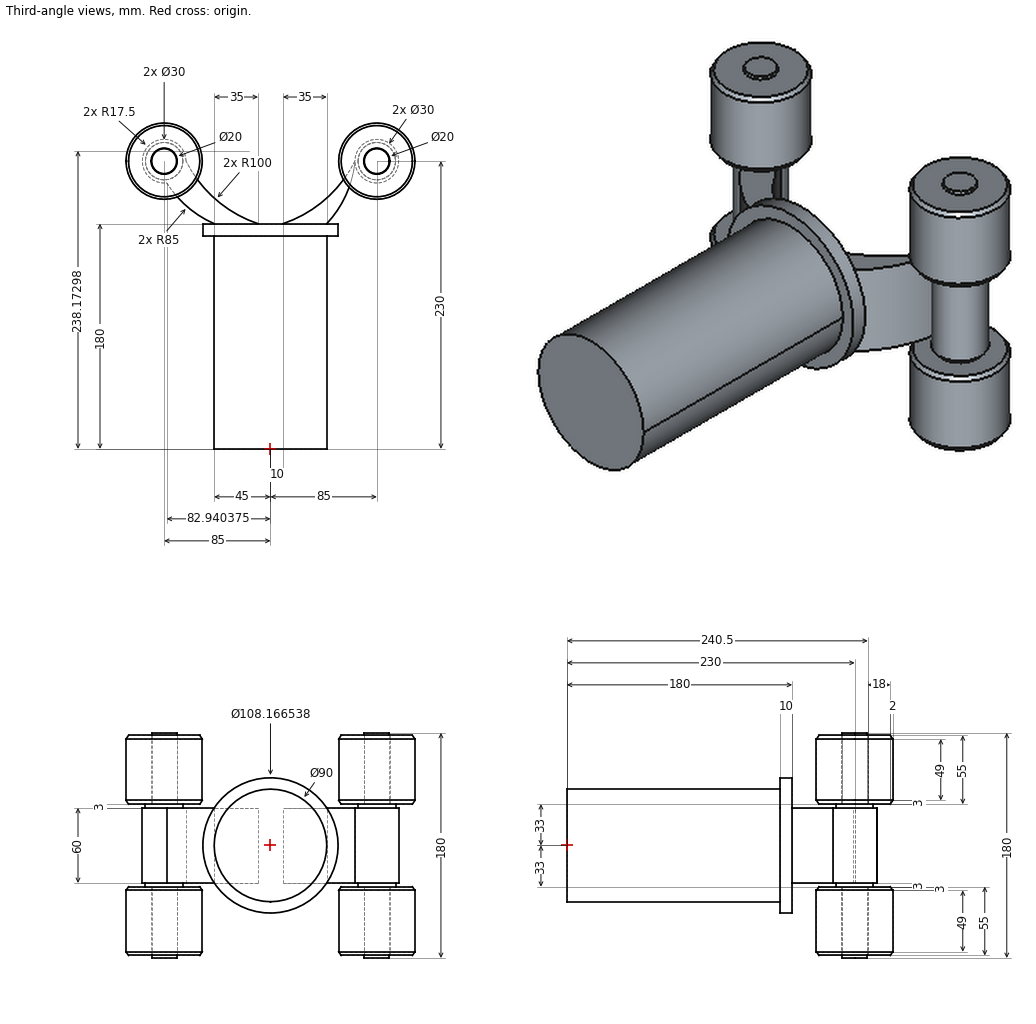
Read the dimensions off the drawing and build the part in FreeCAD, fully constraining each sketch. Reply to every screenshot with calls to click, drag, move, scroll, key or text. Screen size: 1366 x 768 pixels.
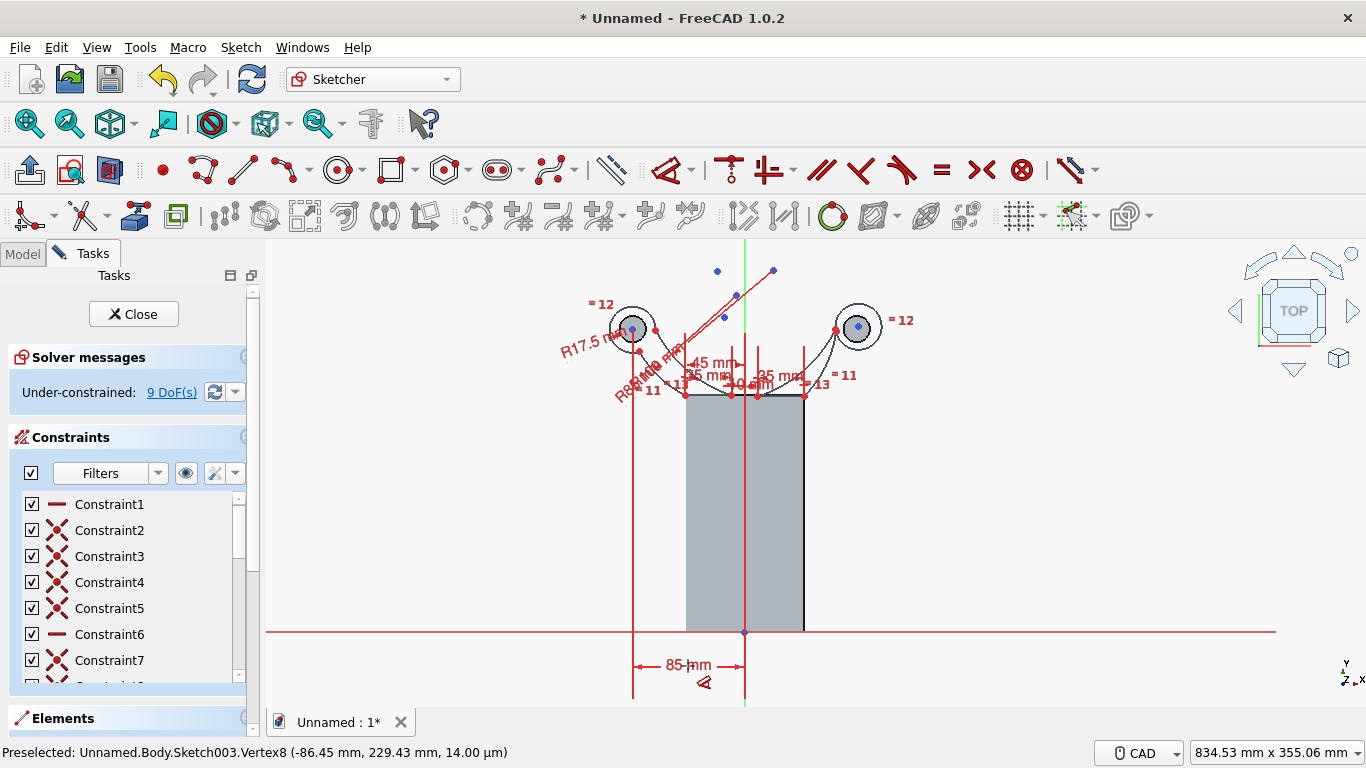
click(859, 327)
click(802, 666)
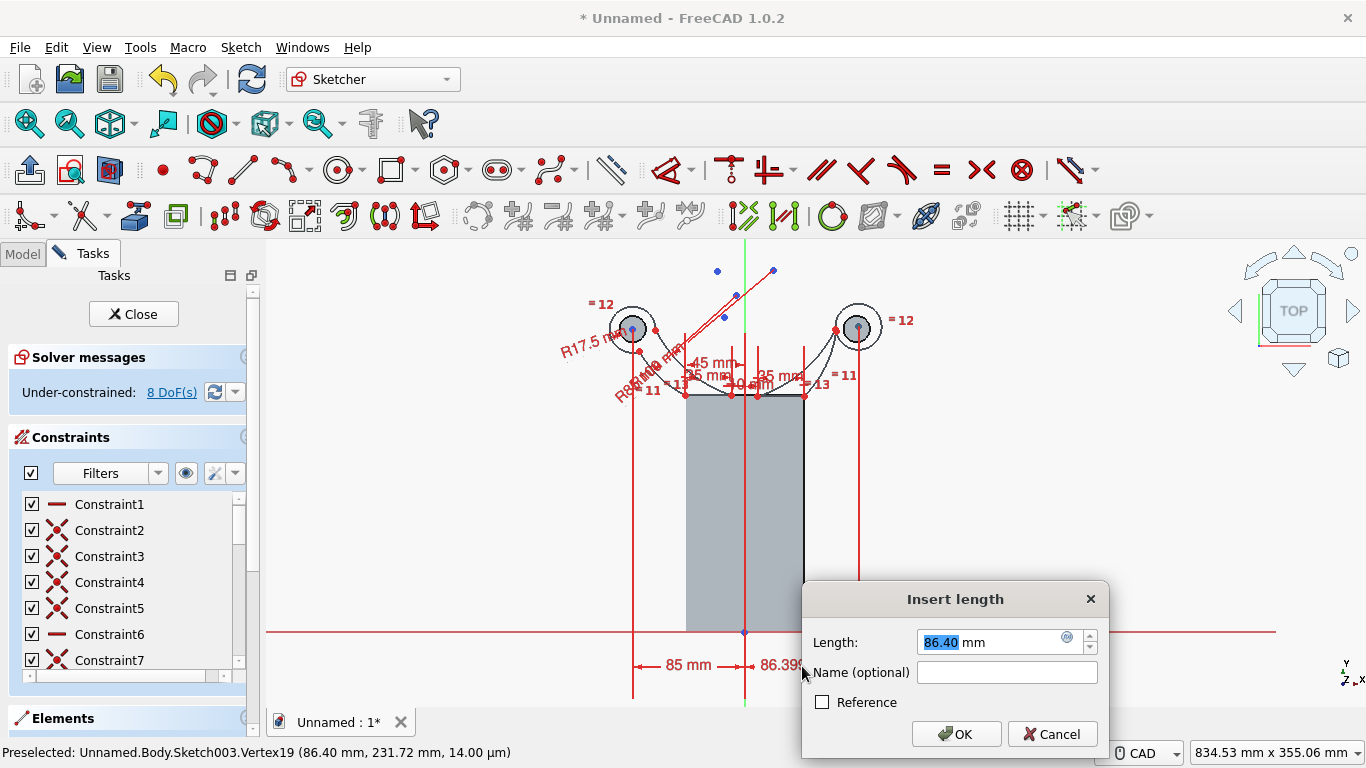
text(85)
key(Return)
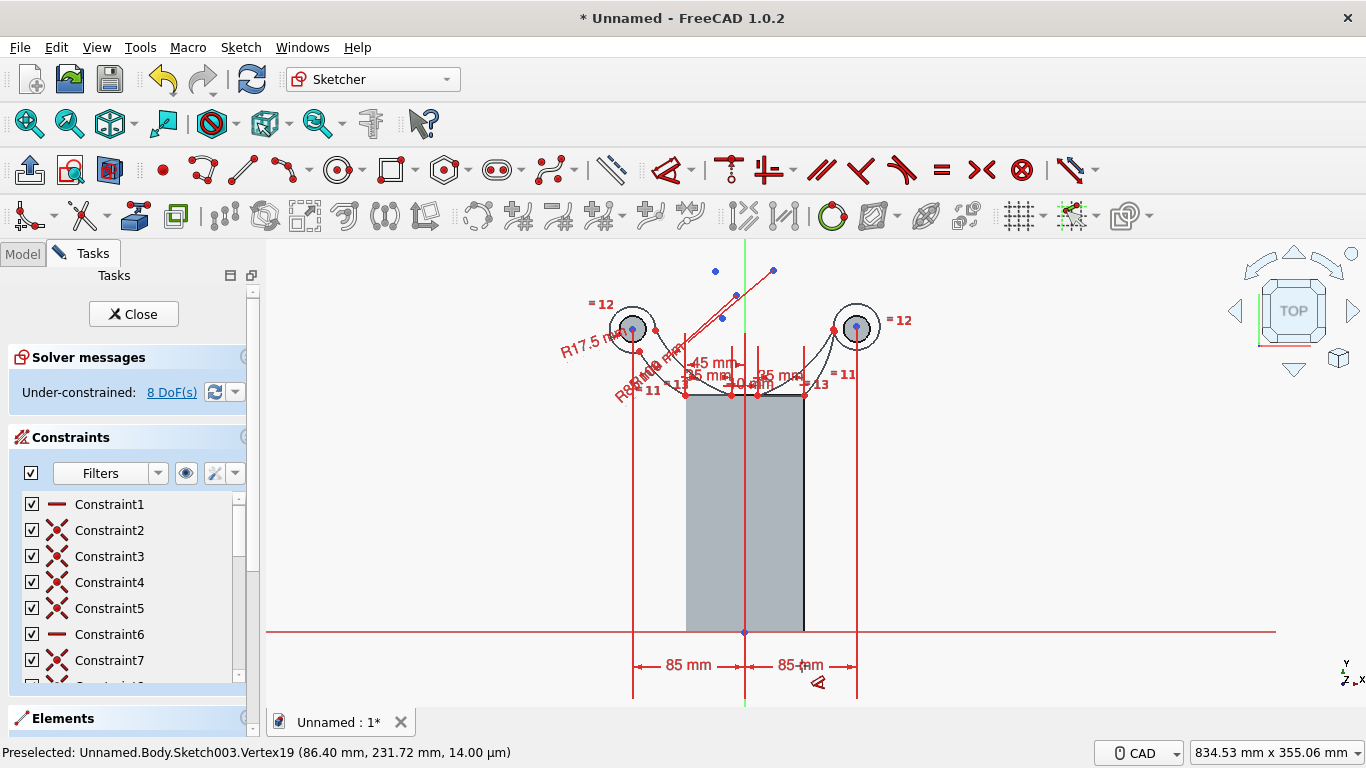
click(685, 395)
click(651, 514)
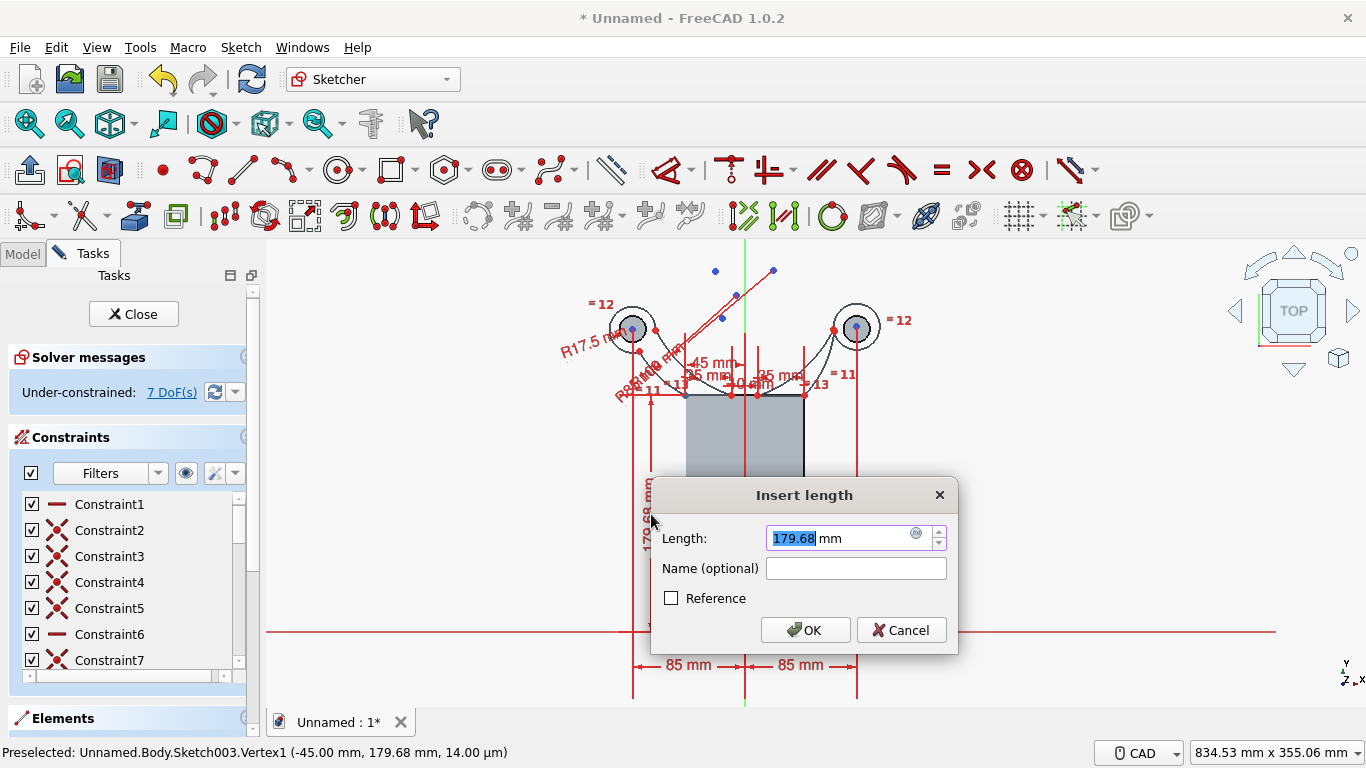
text(180)
key(Return)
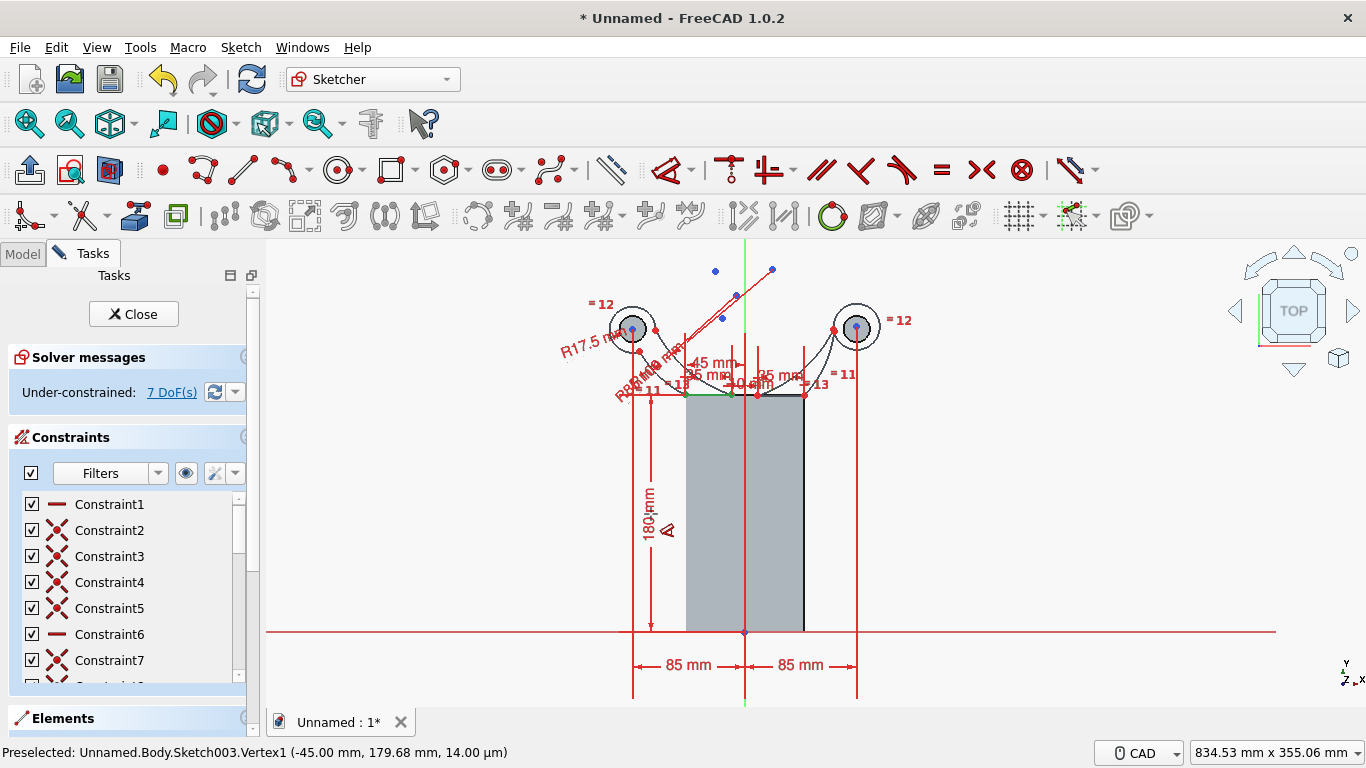
click(656, 330)
click(622, 481)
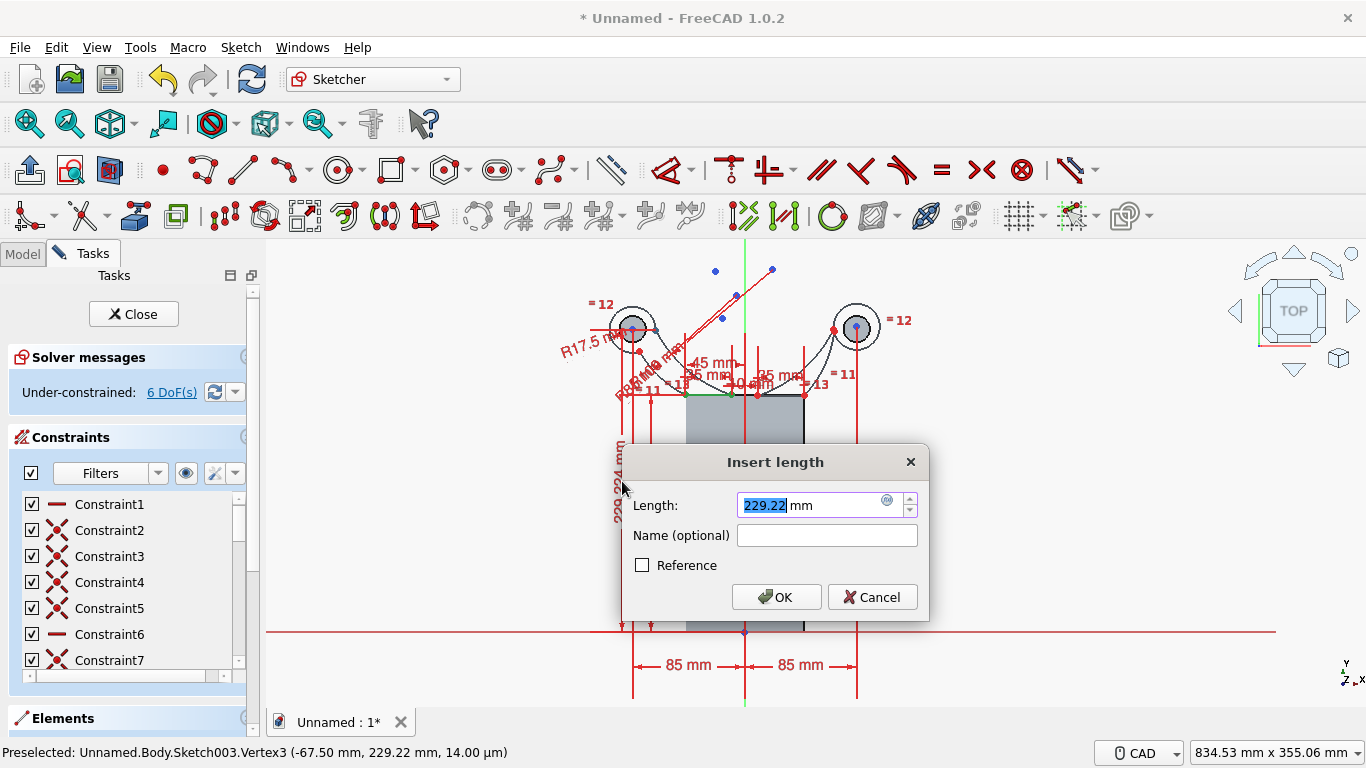
text(230)
key(Return)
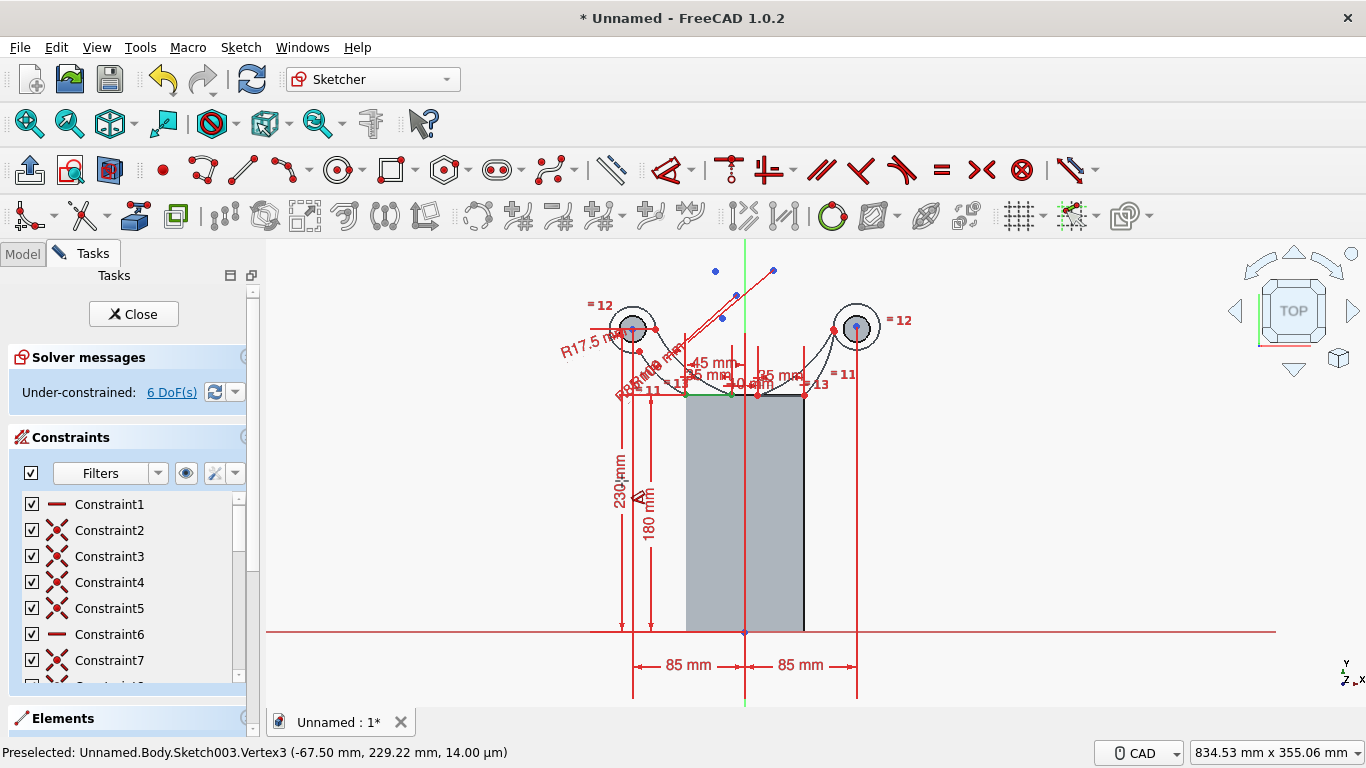
click(758, 396)
click(792, 514)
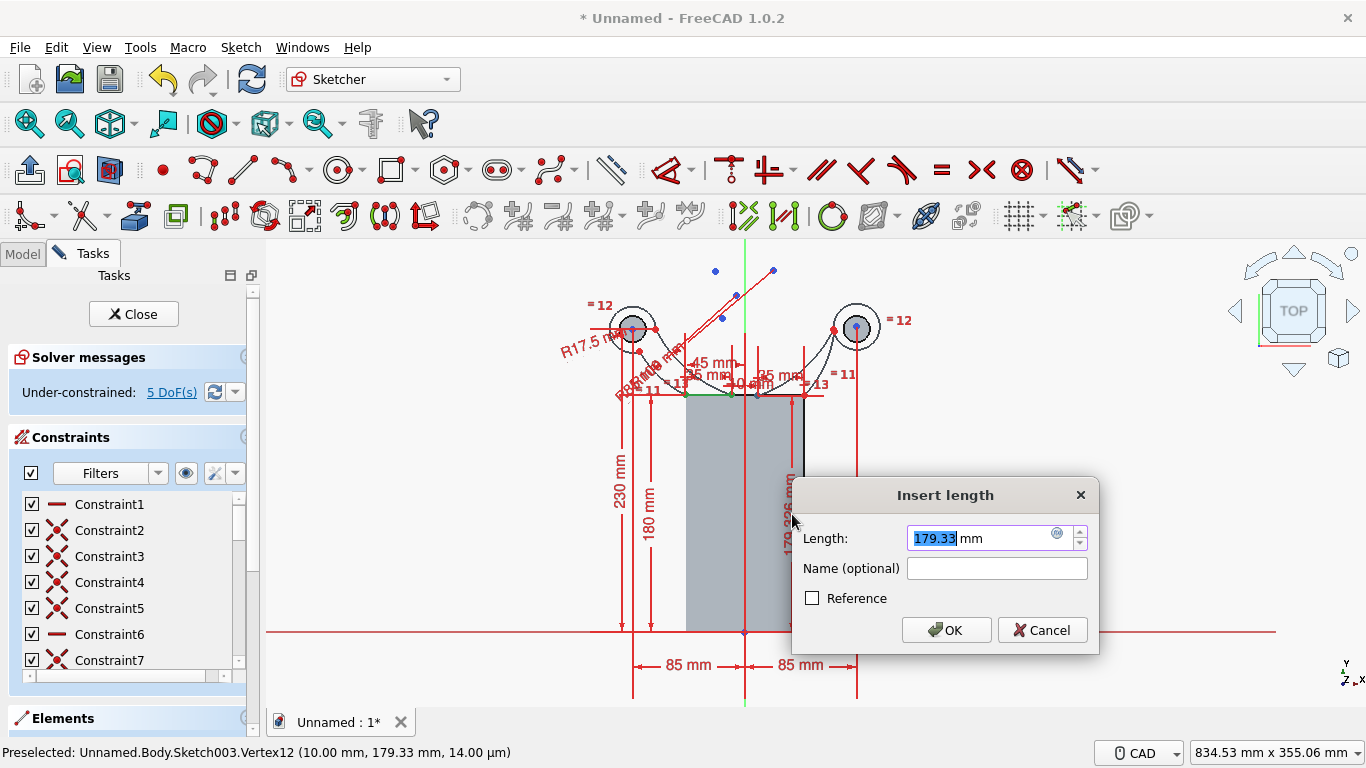
text(180)
key(Return)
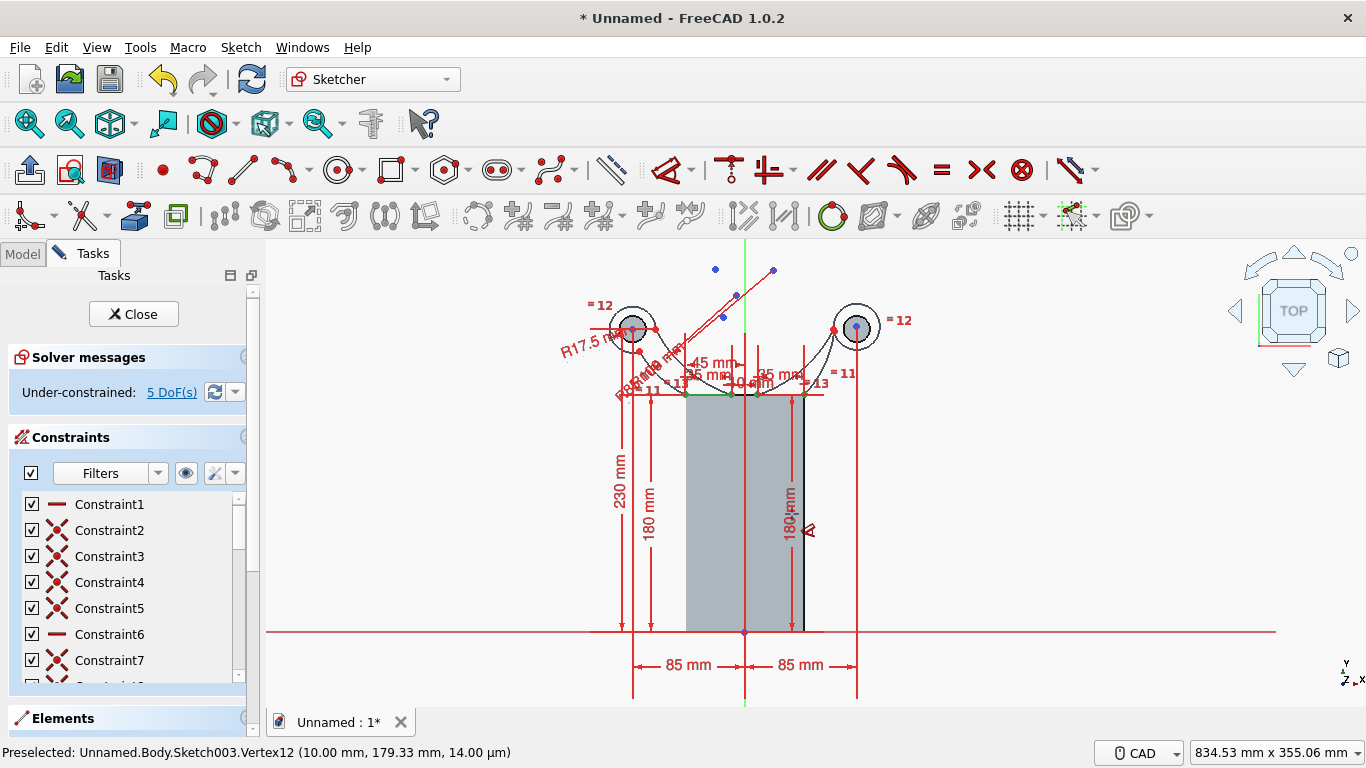
scroll(834, 329, up, 8)